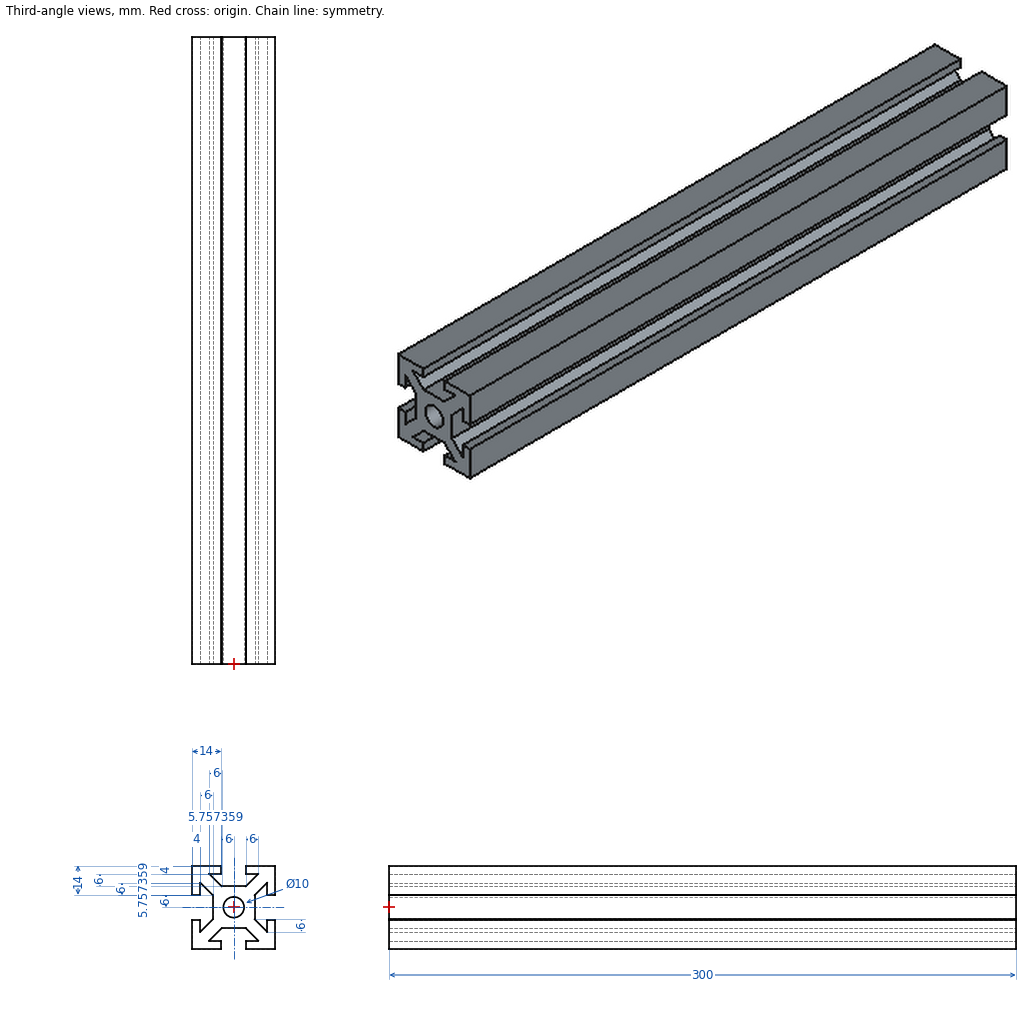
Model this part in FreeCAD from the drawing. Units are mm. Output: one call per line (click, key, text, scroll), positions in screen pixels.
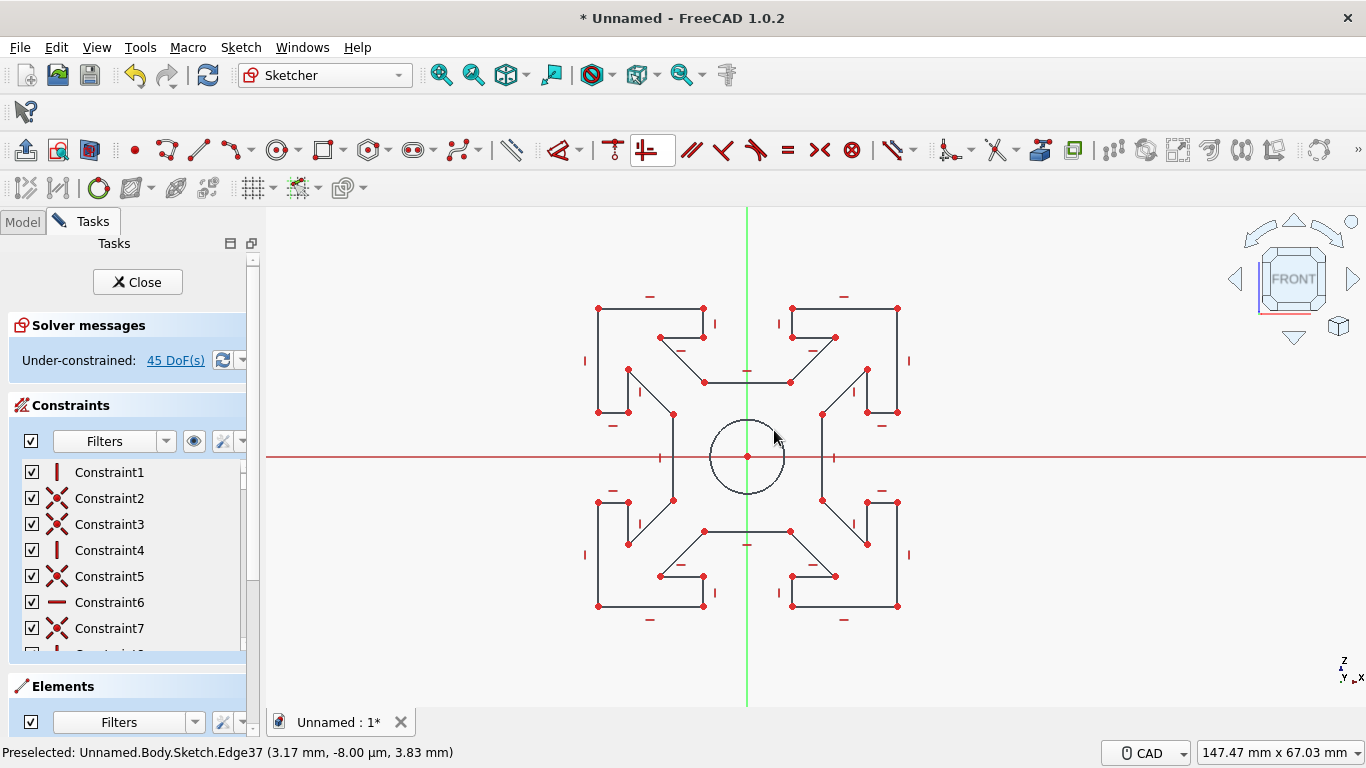
click(660, 338)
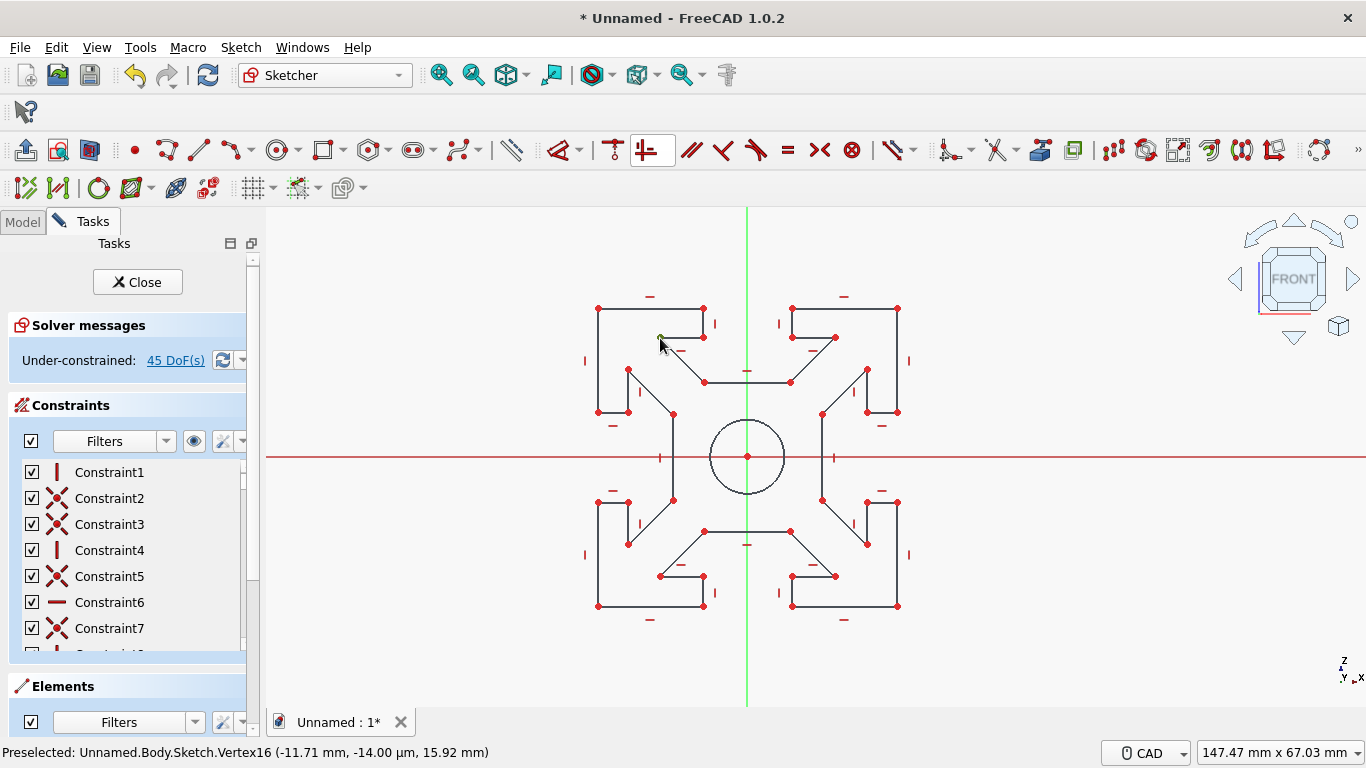
click(835, 338)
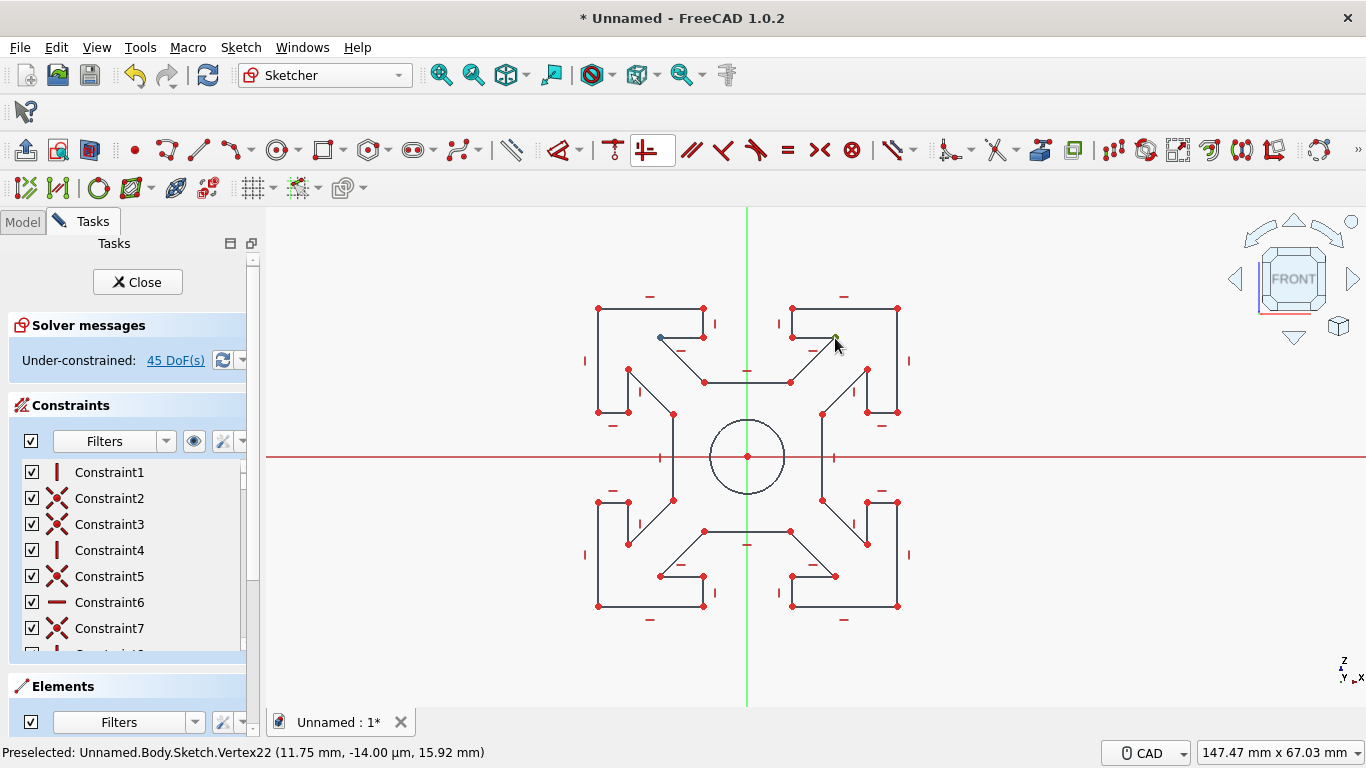
click(747, 647)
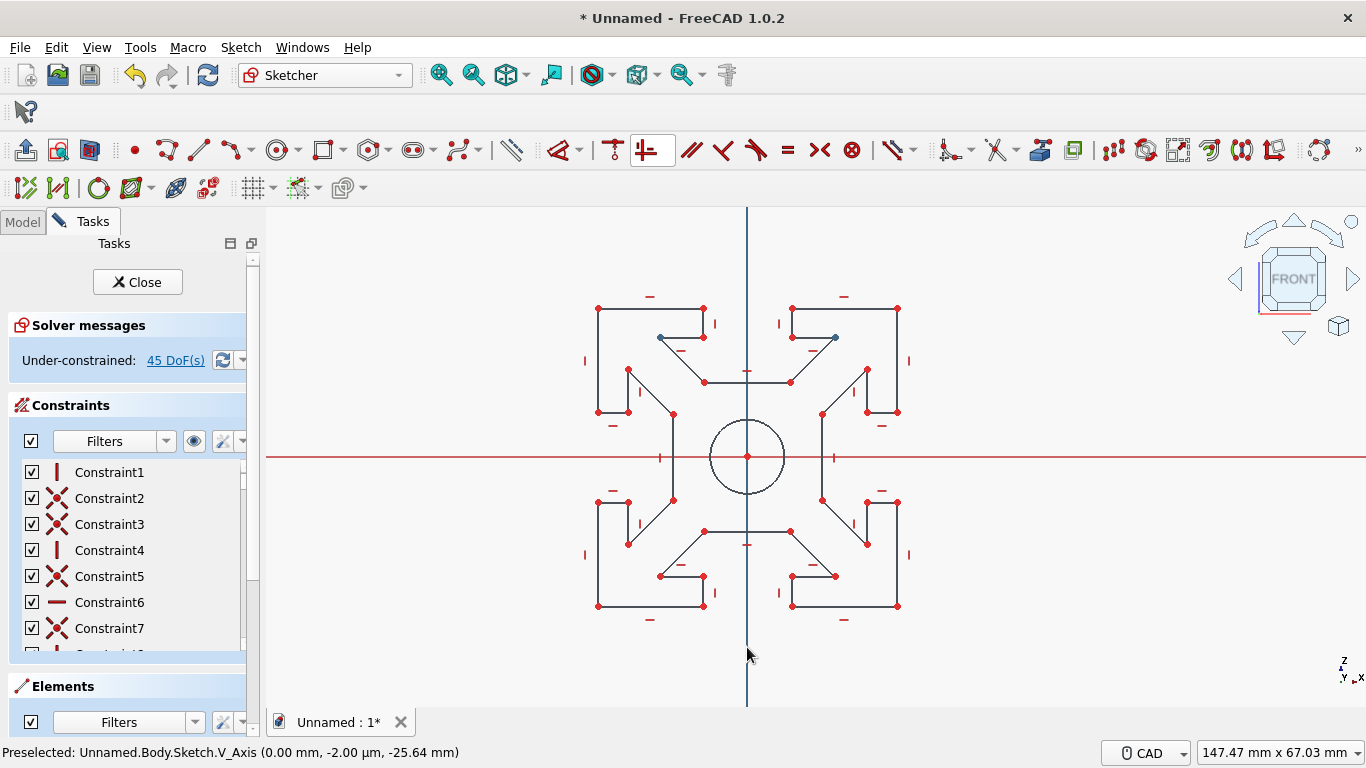
click(820, 150)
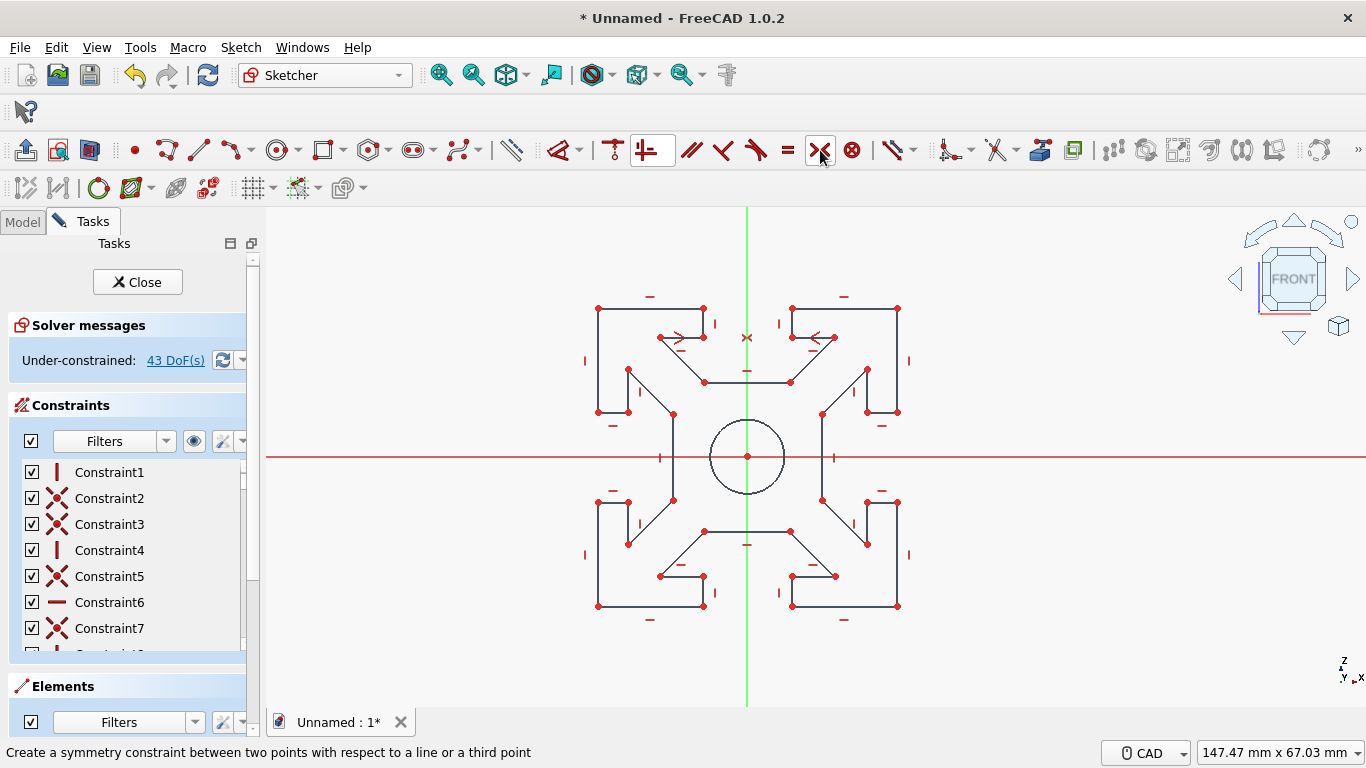
click(703, 309)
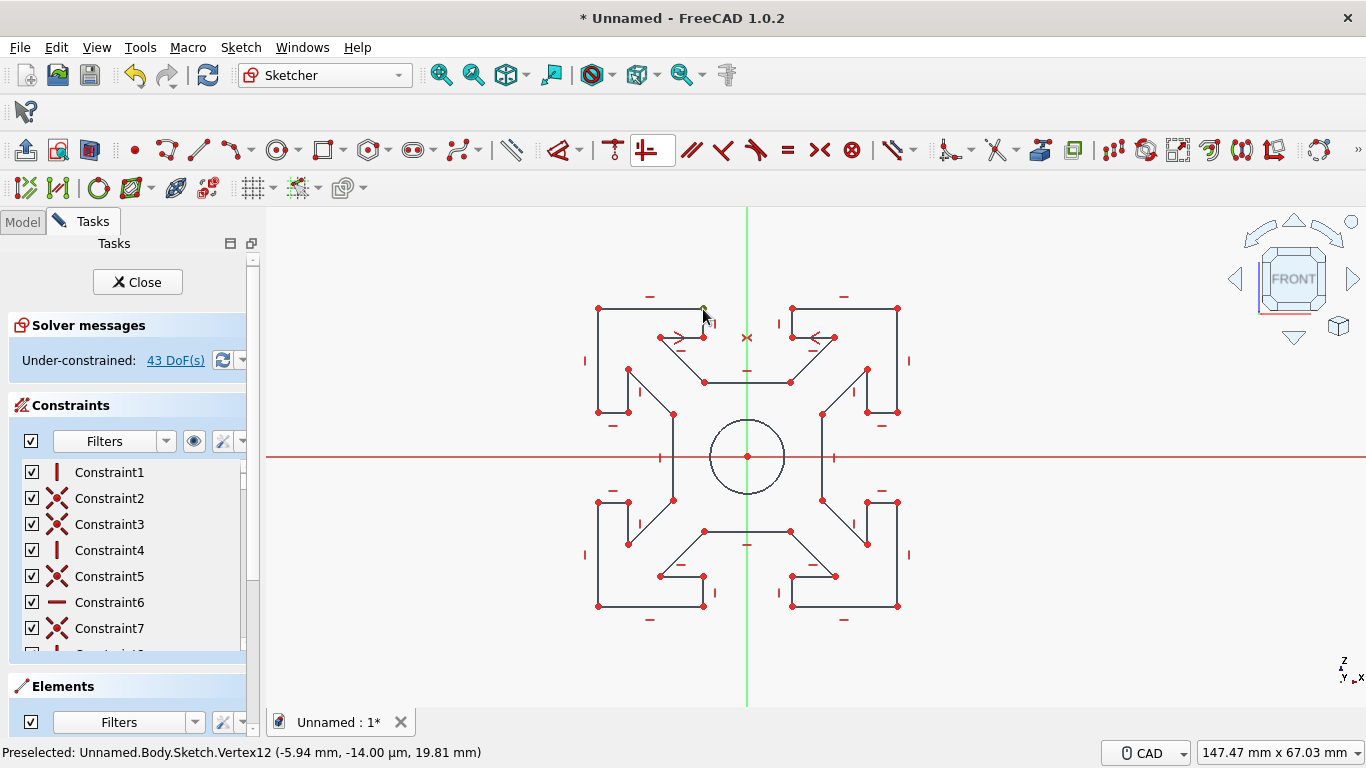
click(792, 309)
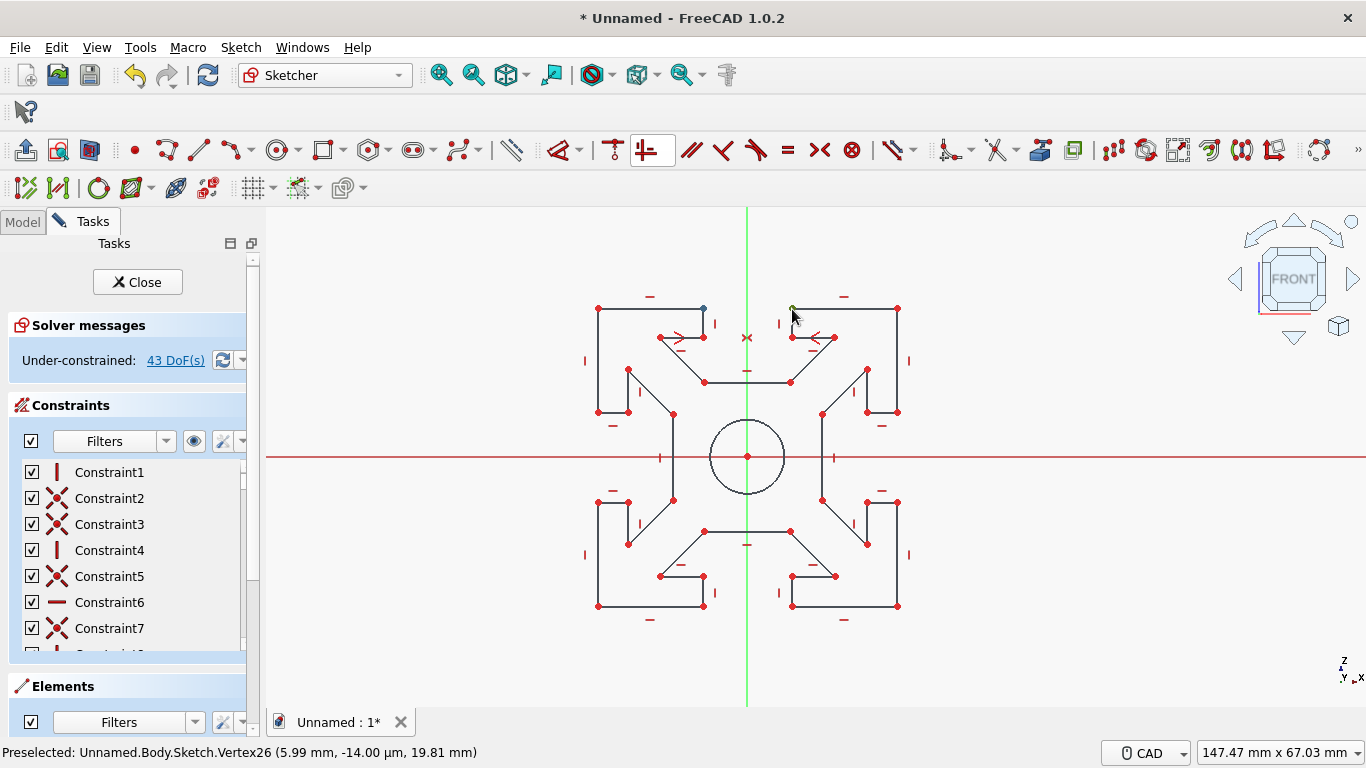
click(747, 647)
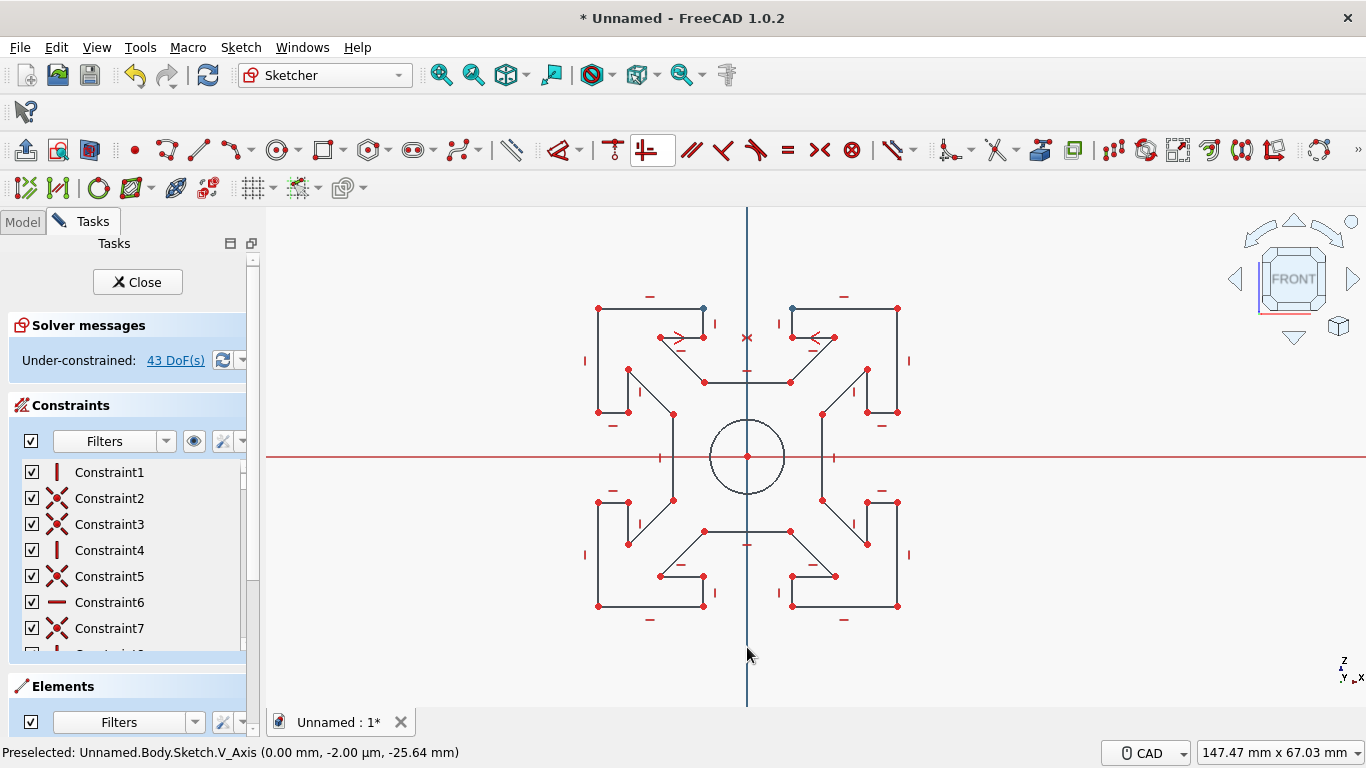
click(820, 150)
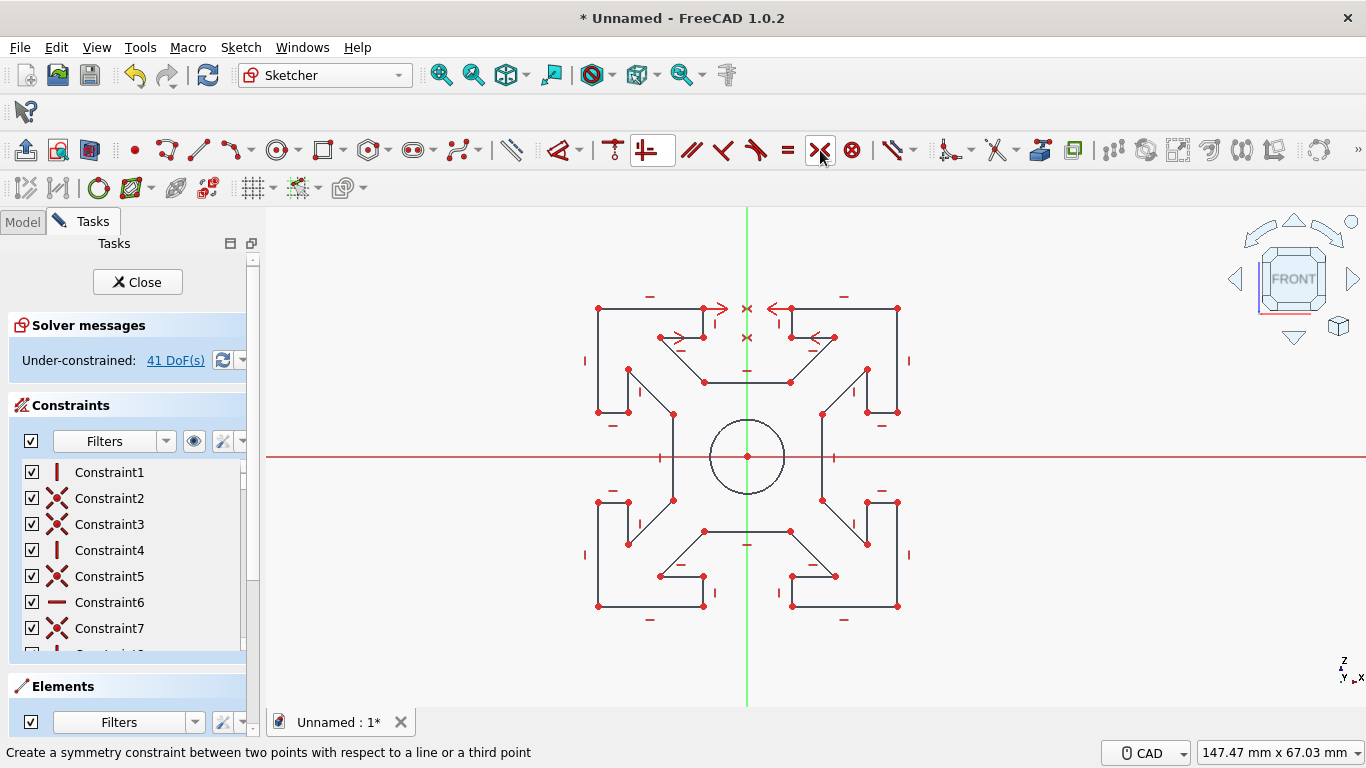
click(598, 413)